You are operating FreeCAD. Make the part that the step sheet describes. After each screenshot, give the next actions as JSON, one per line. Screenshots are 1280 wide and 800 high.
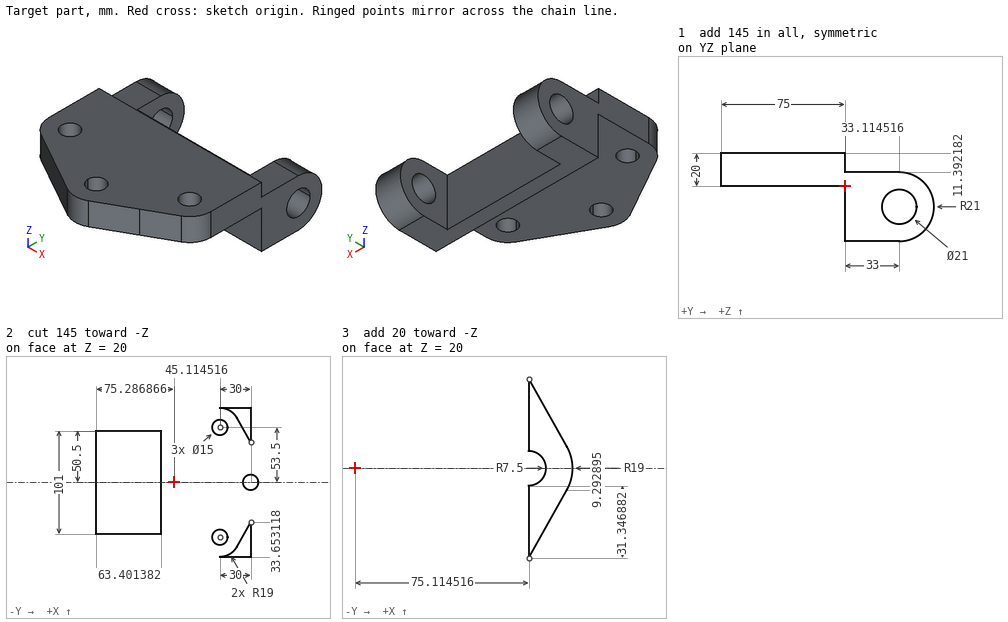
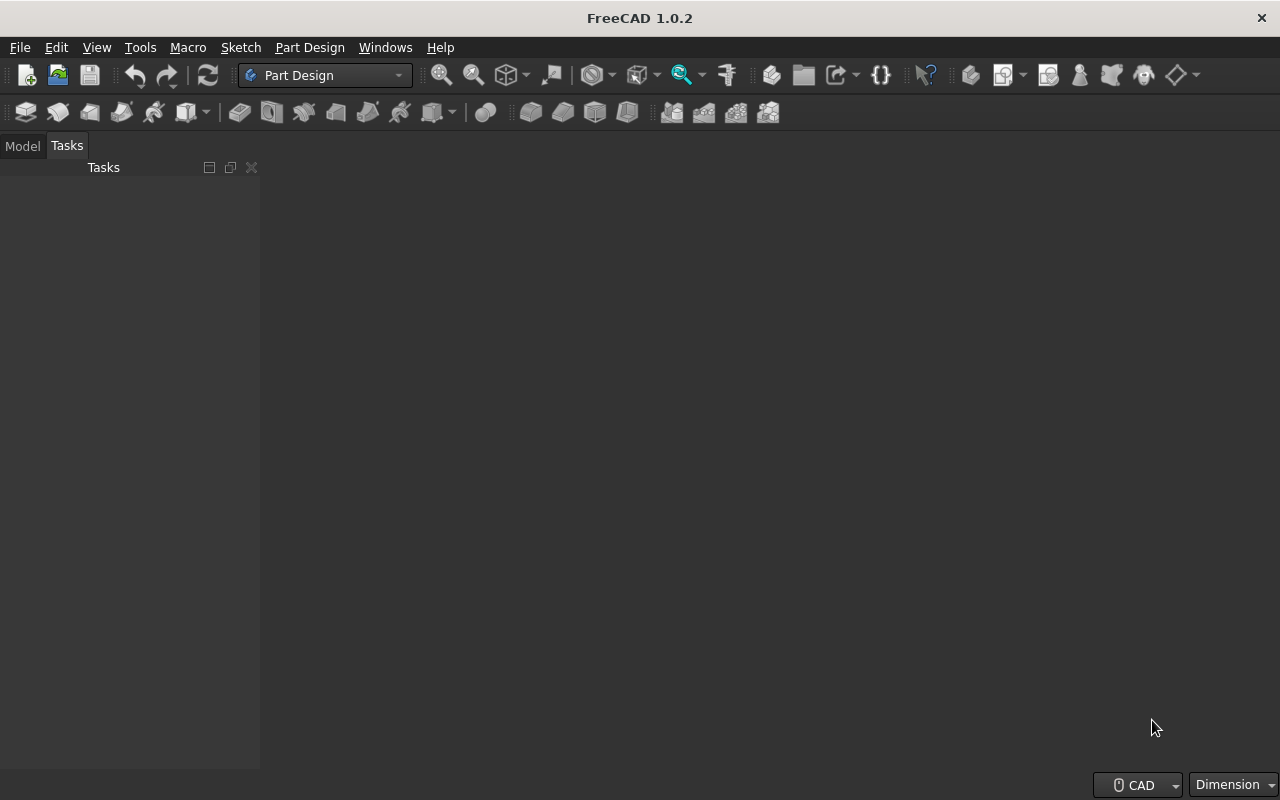
{"action": "left_click", "coordinate": [26, 76]}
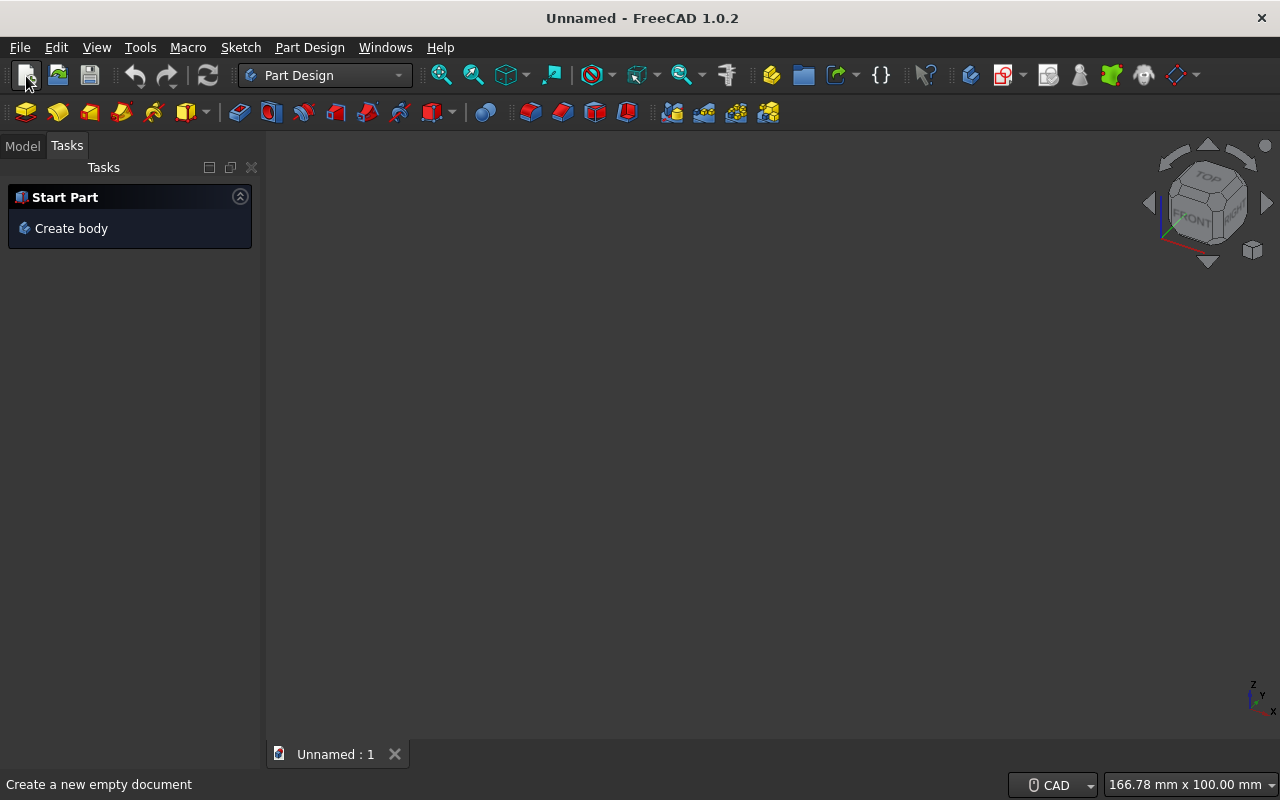
{"action": "left_click", "coordinate": [1004, 76]}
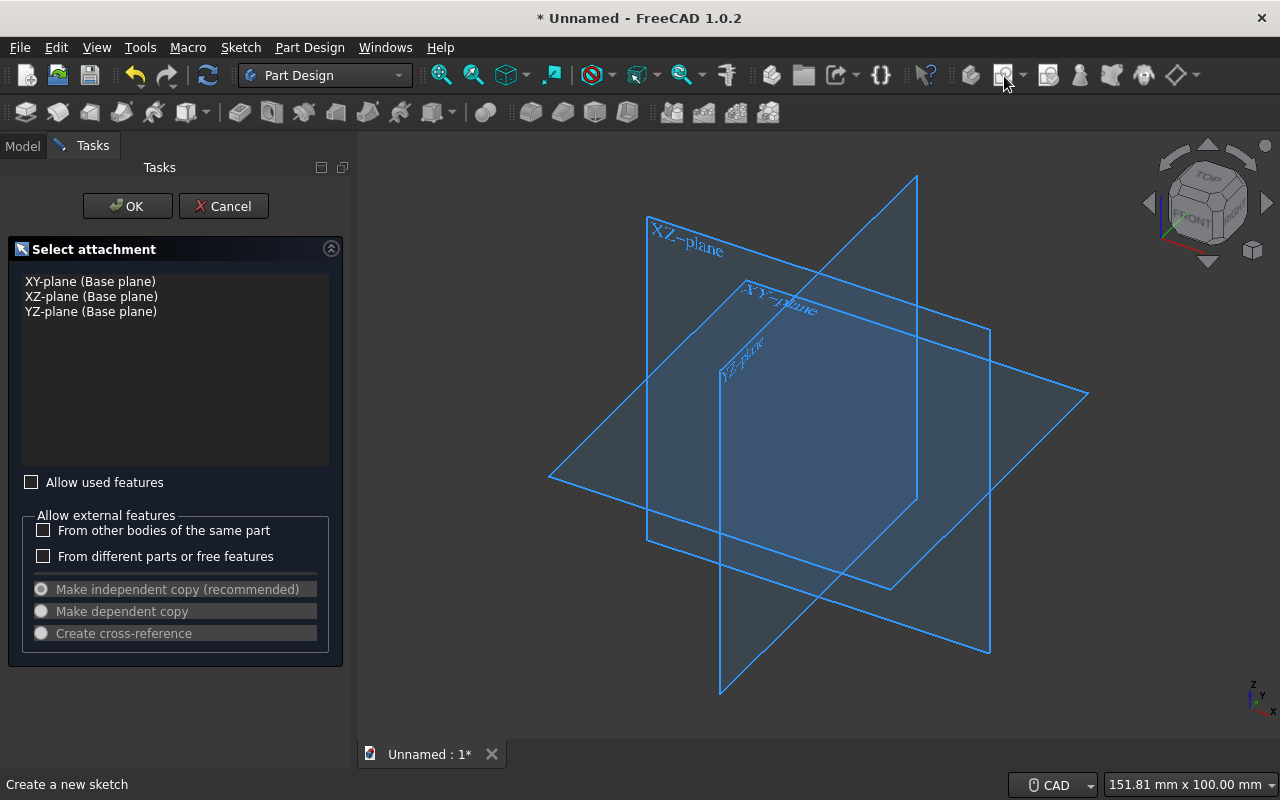
{"action": "left_click", "coordinate": [82, 312]}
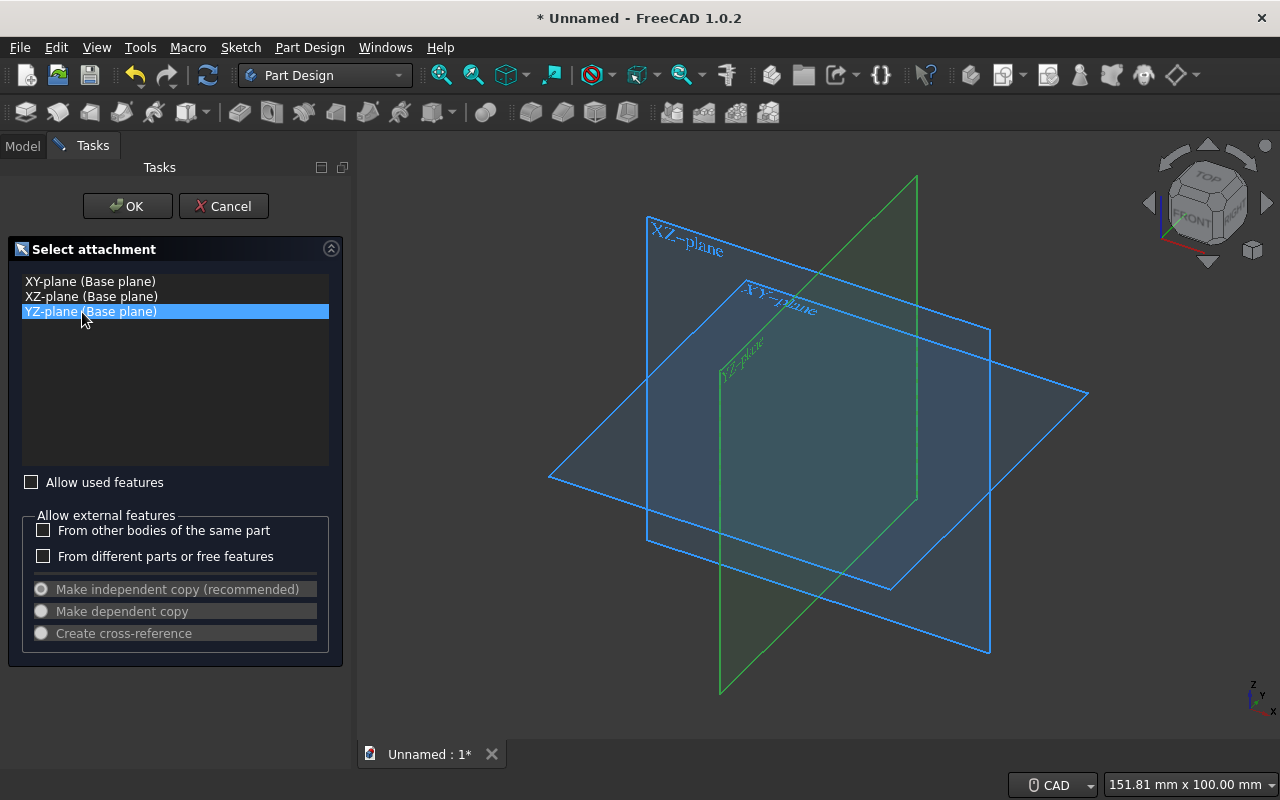
{"action": "left_click", "coordinate": [128, 206]}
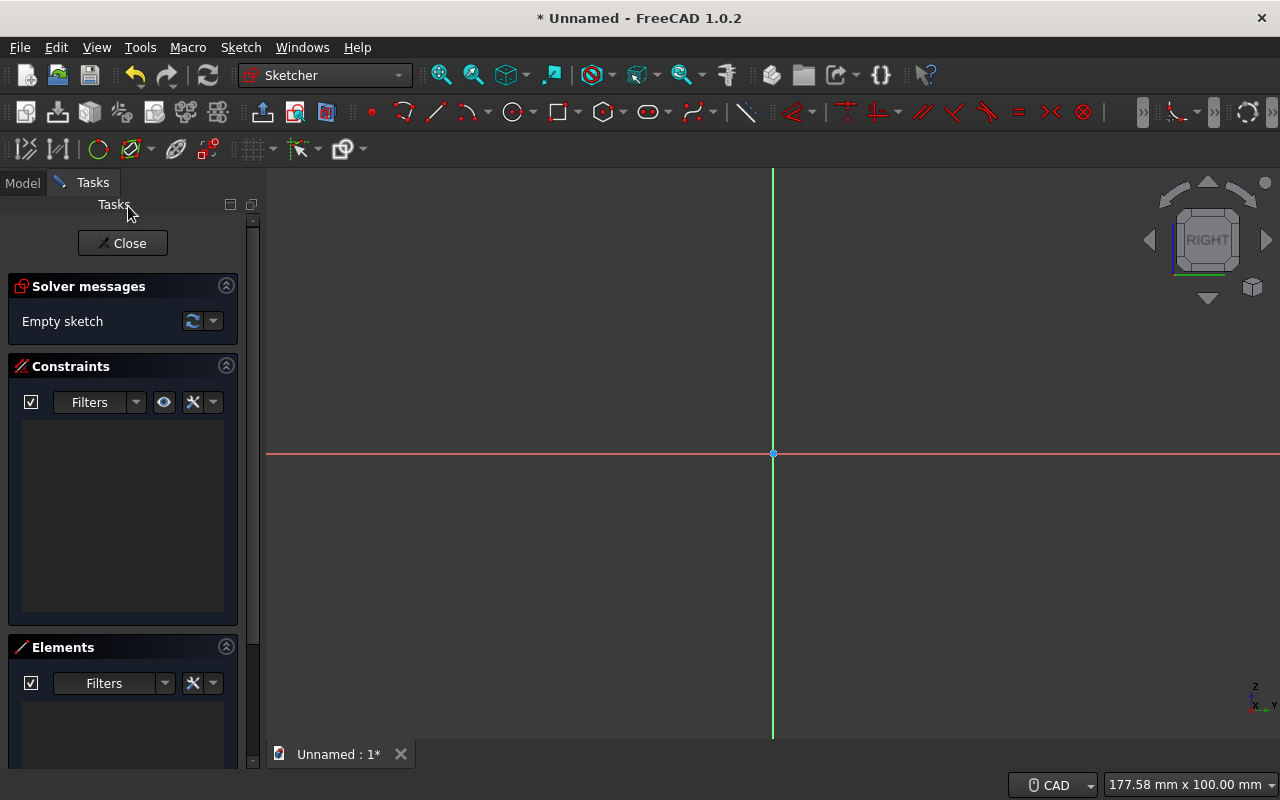
{"action": "left_click", "coordinate": [404, 112]}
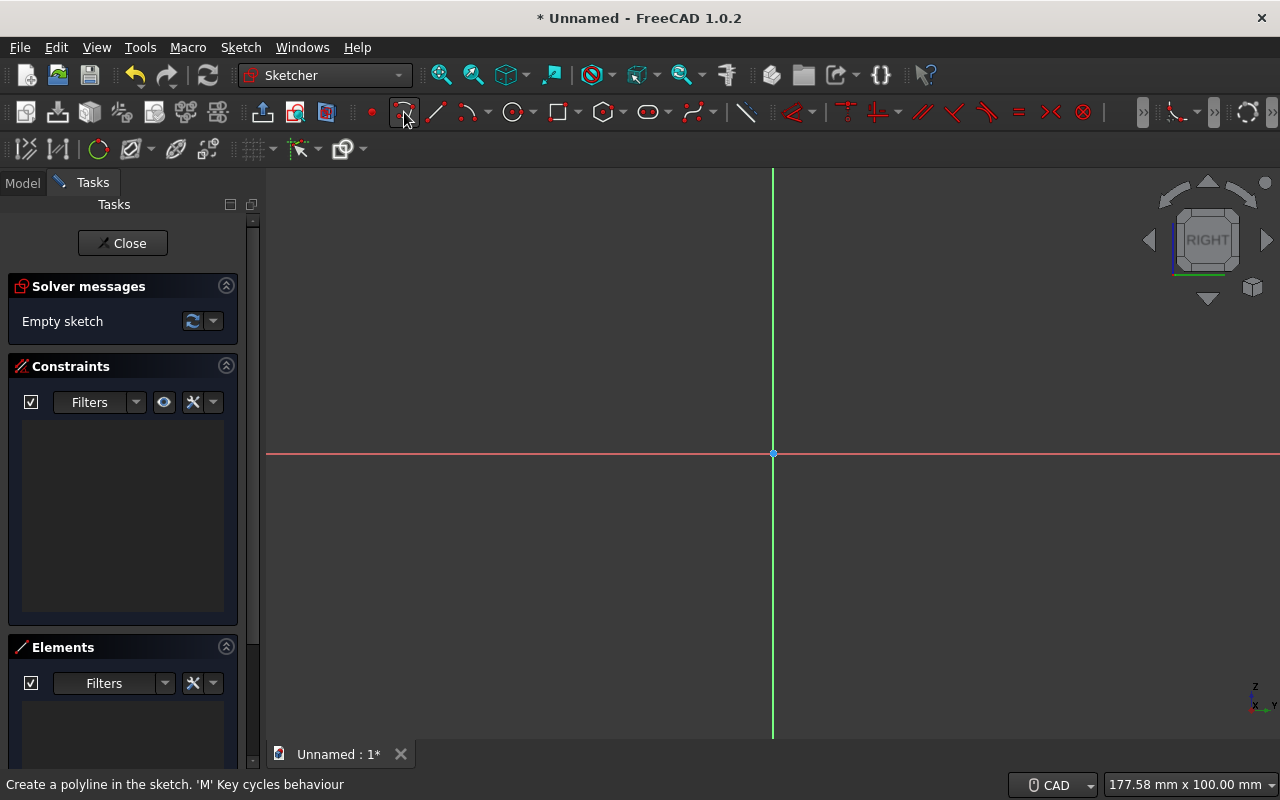
{"action": "left_click", "coordinate": [961, 404]}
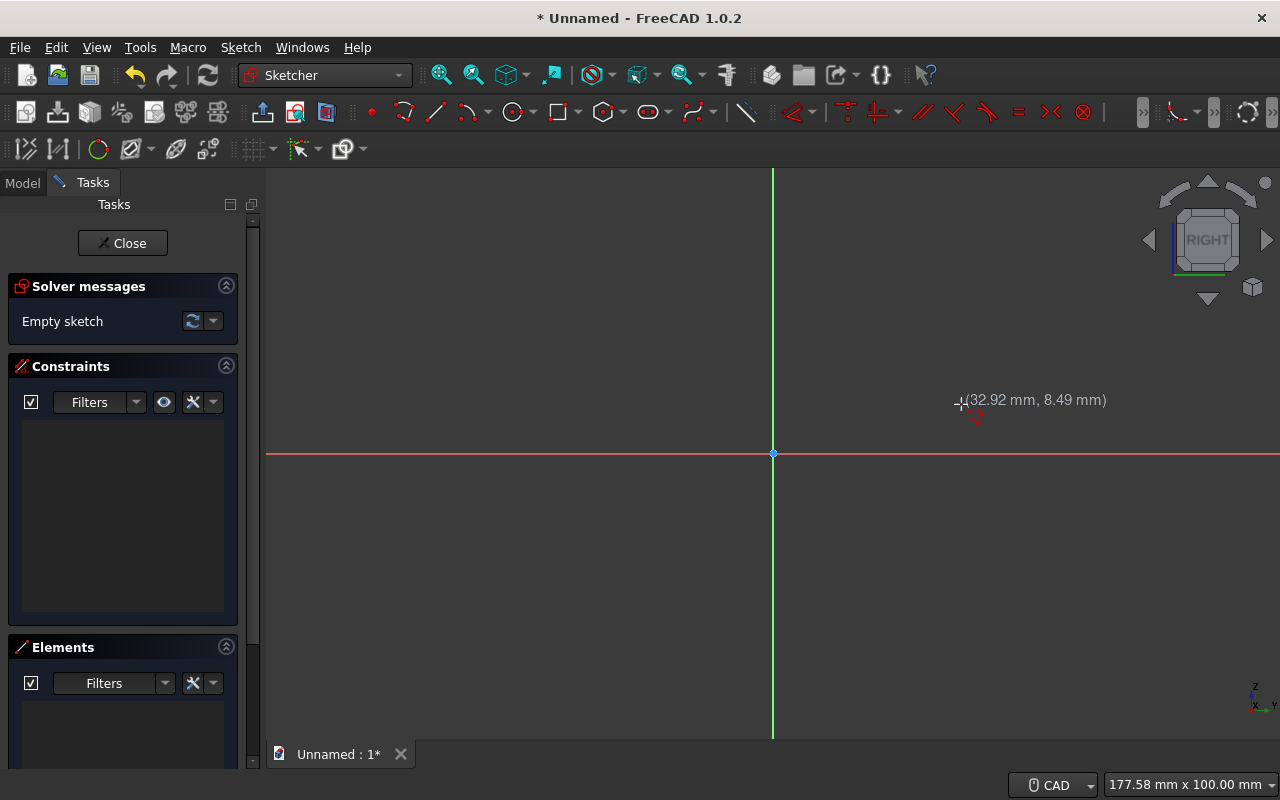
{"action": "scroll", "coordinate": [772, 404], "scroll_direction": "up", "scroll_amount": 16}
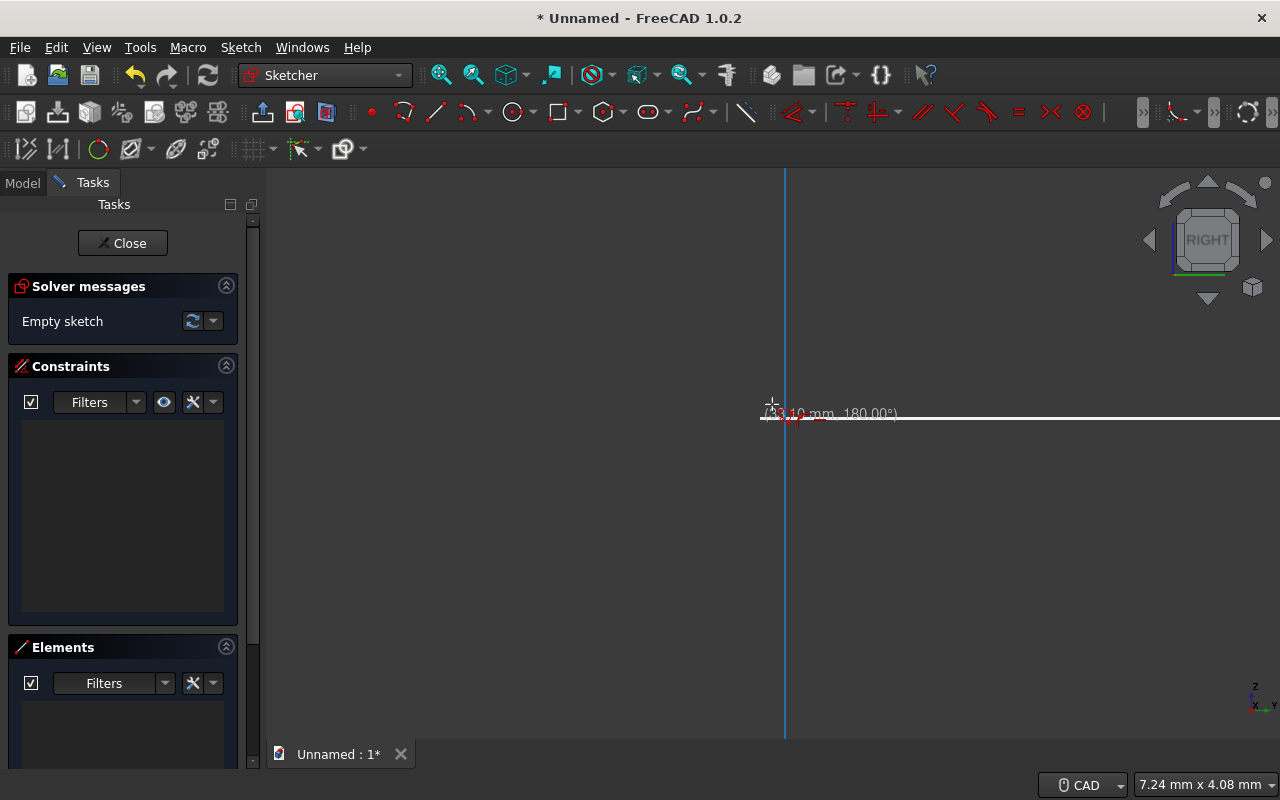
{"action": "left_click", "coordinate": [769, 394]}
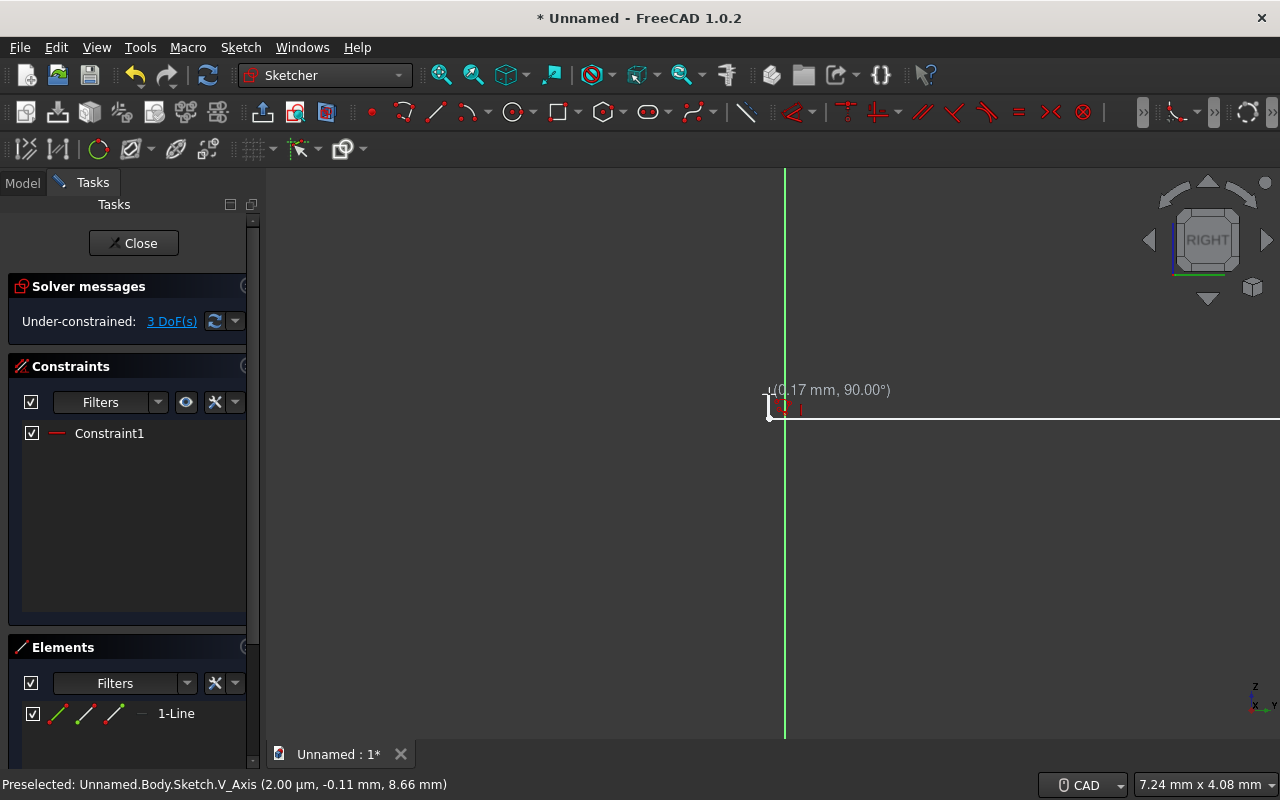
{"action": "scroll", "coordinate": [764, 365], "scroll_direction": "down", "scroll_amount": 16}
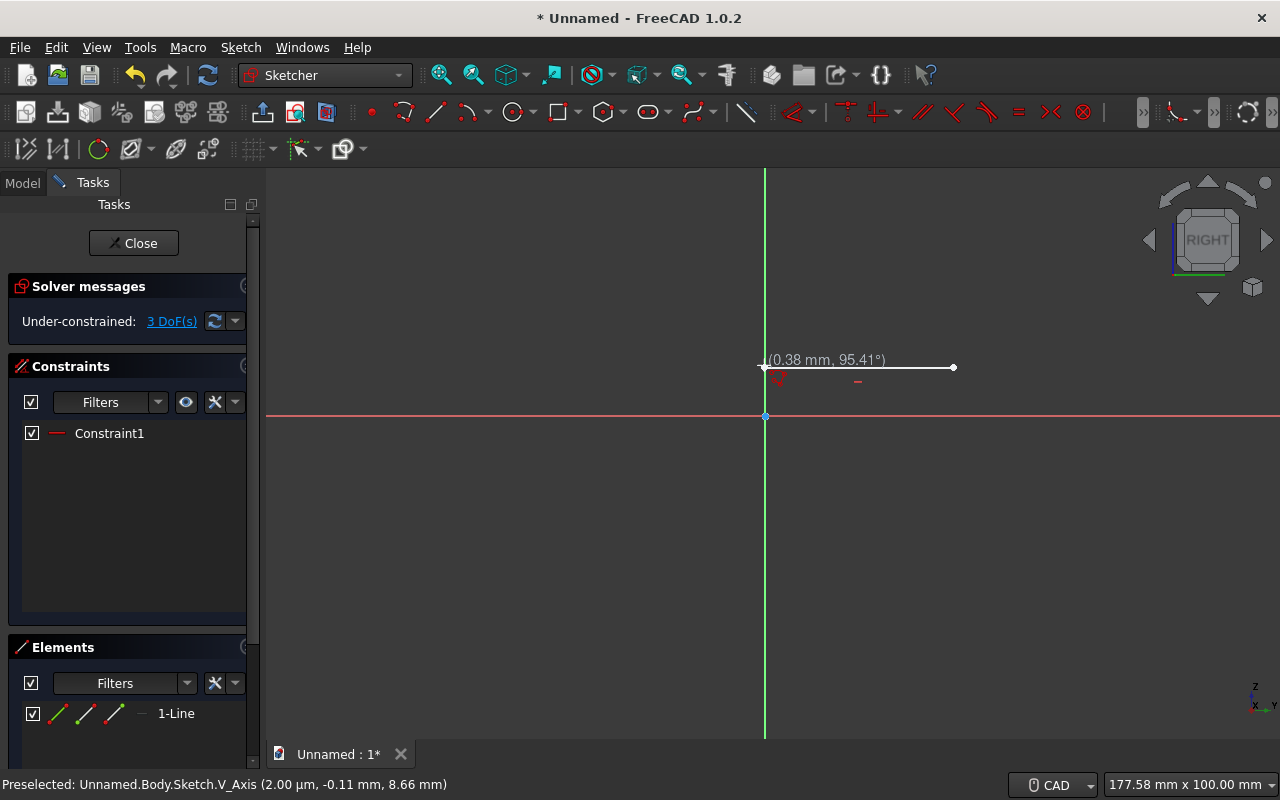
{"action": "scroll", "coordinate": [765, 302], "scroll_direction": "up", "scroll_amount": 16}